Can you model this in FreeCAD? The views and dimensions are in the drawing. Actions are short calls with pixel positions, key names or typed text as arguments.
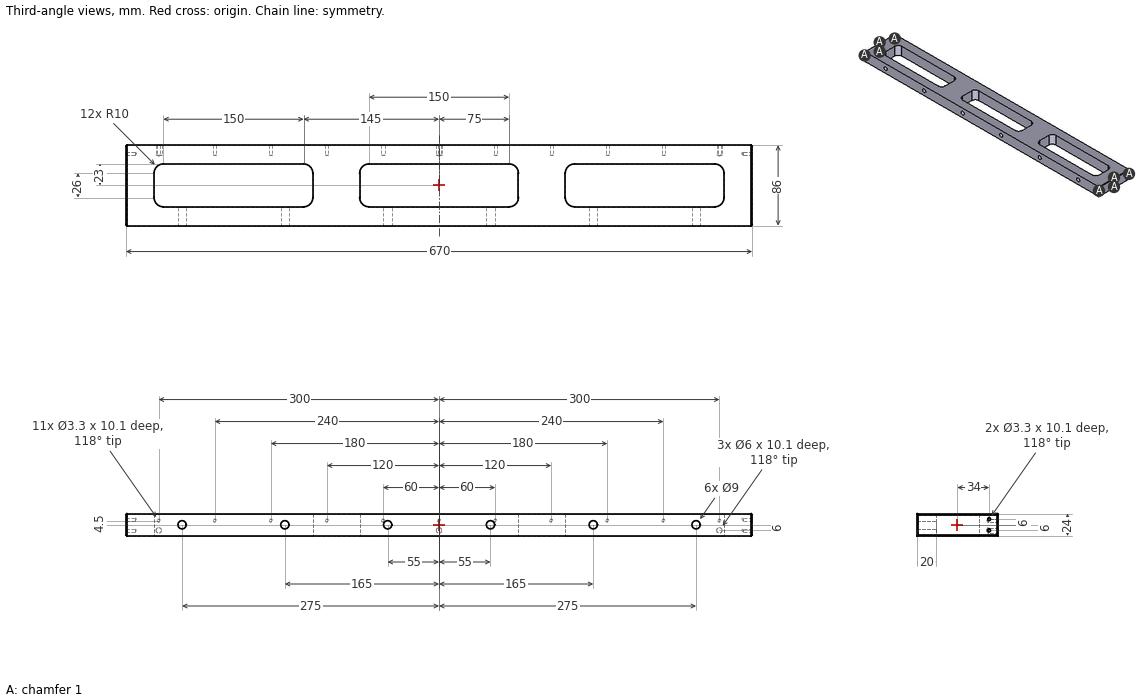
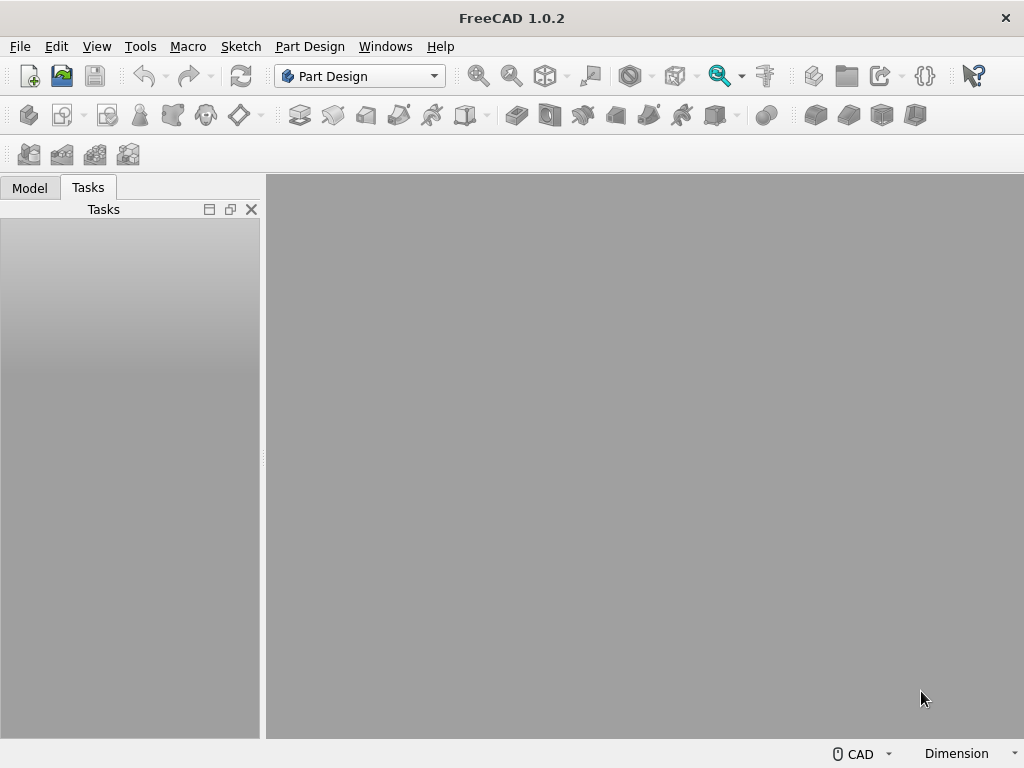
key(ctrl+n)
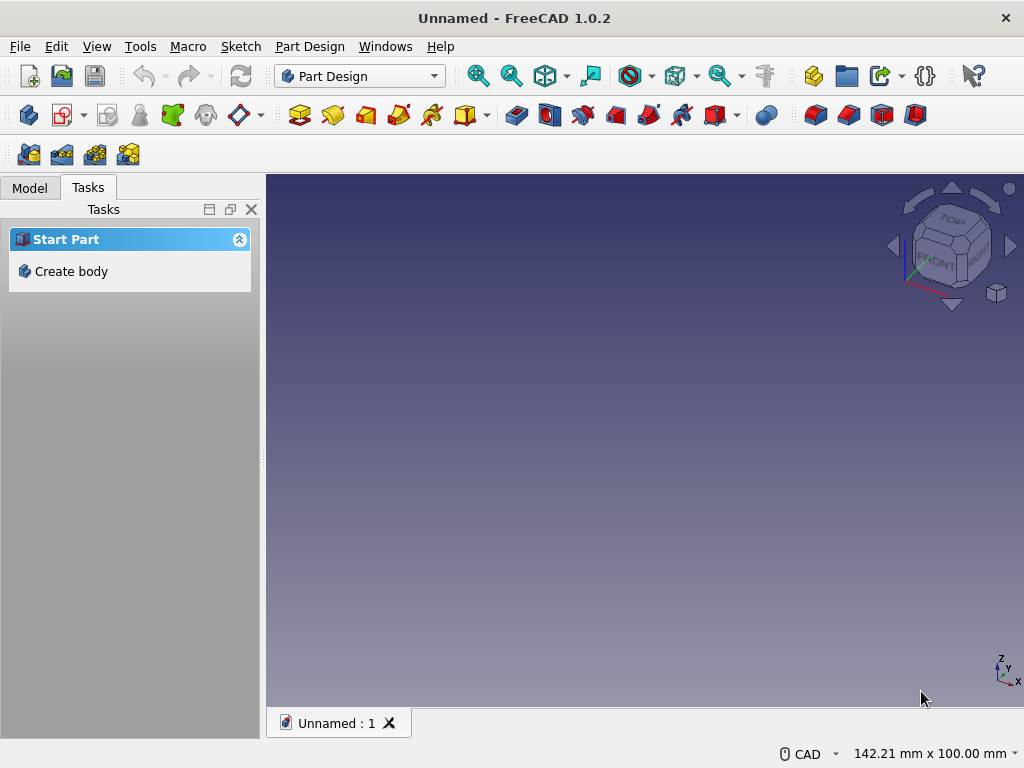
click(62, 116)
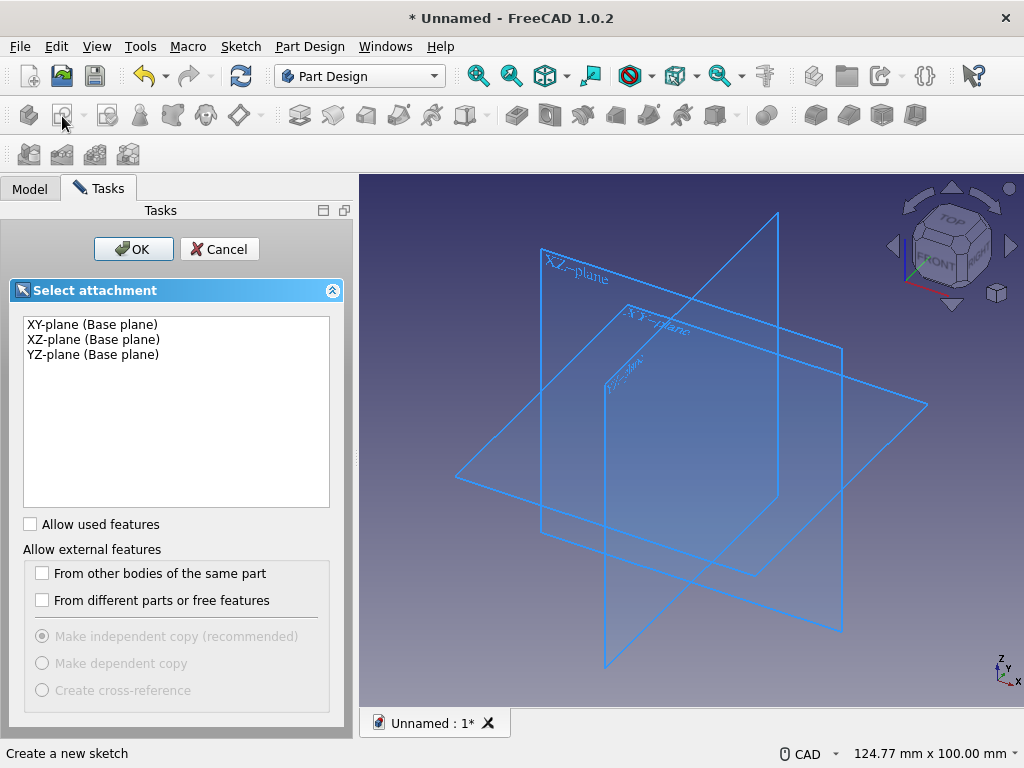
click(84, 324)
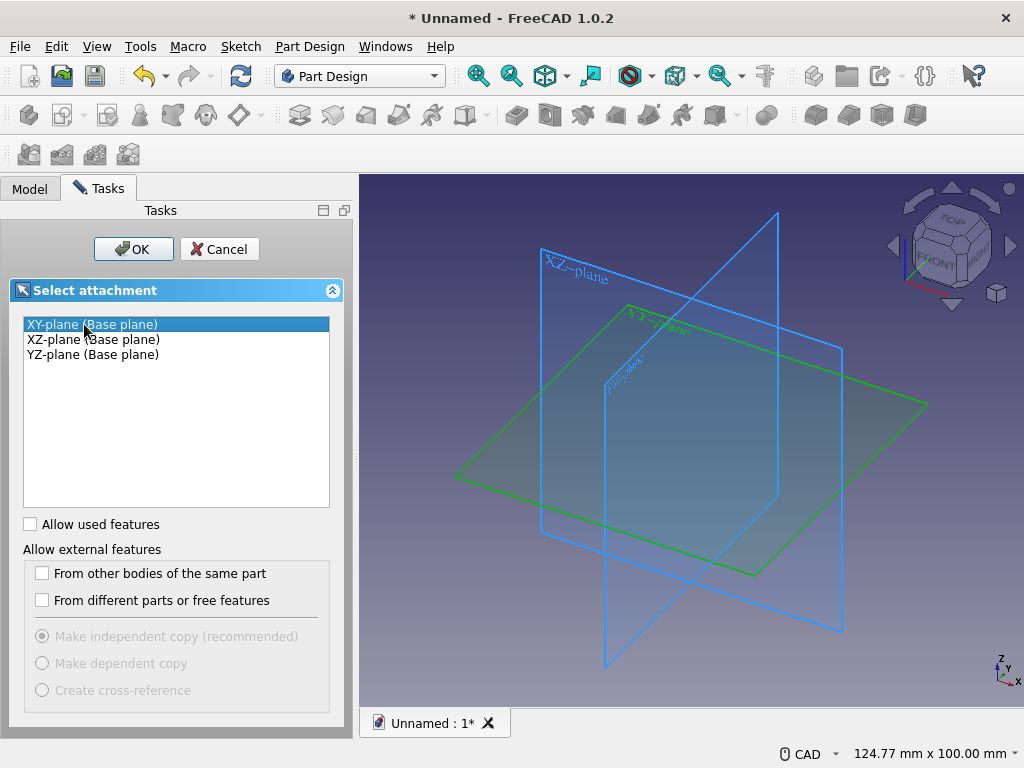
click(134, 249)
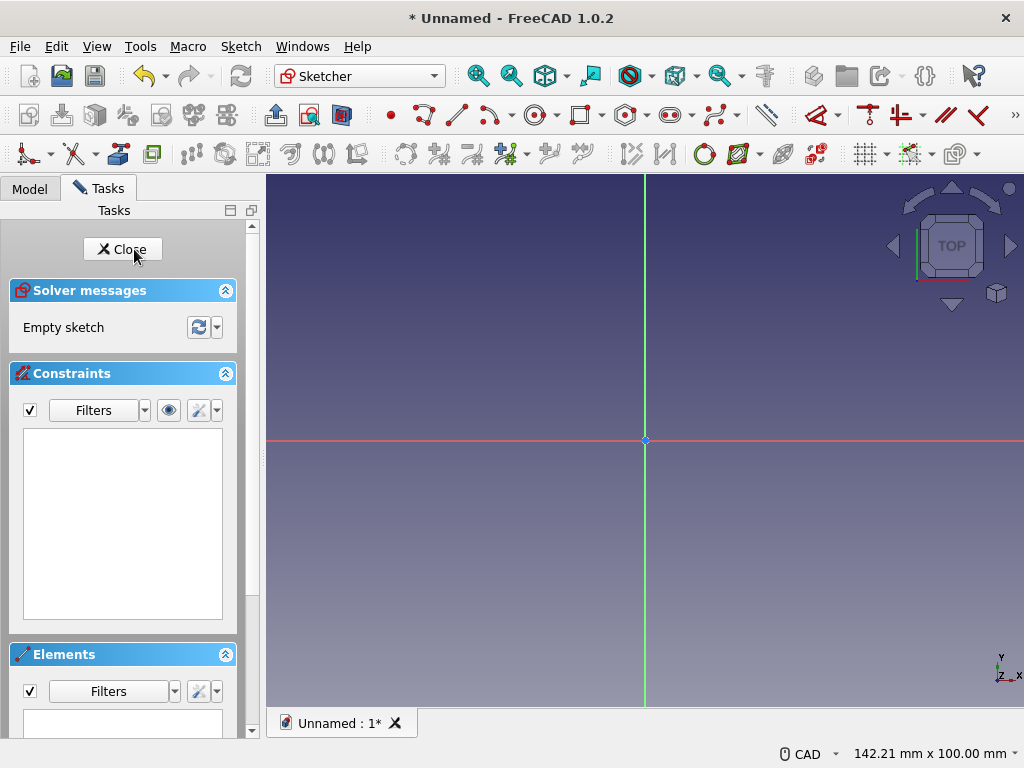
scroll(568, 441, down, 11)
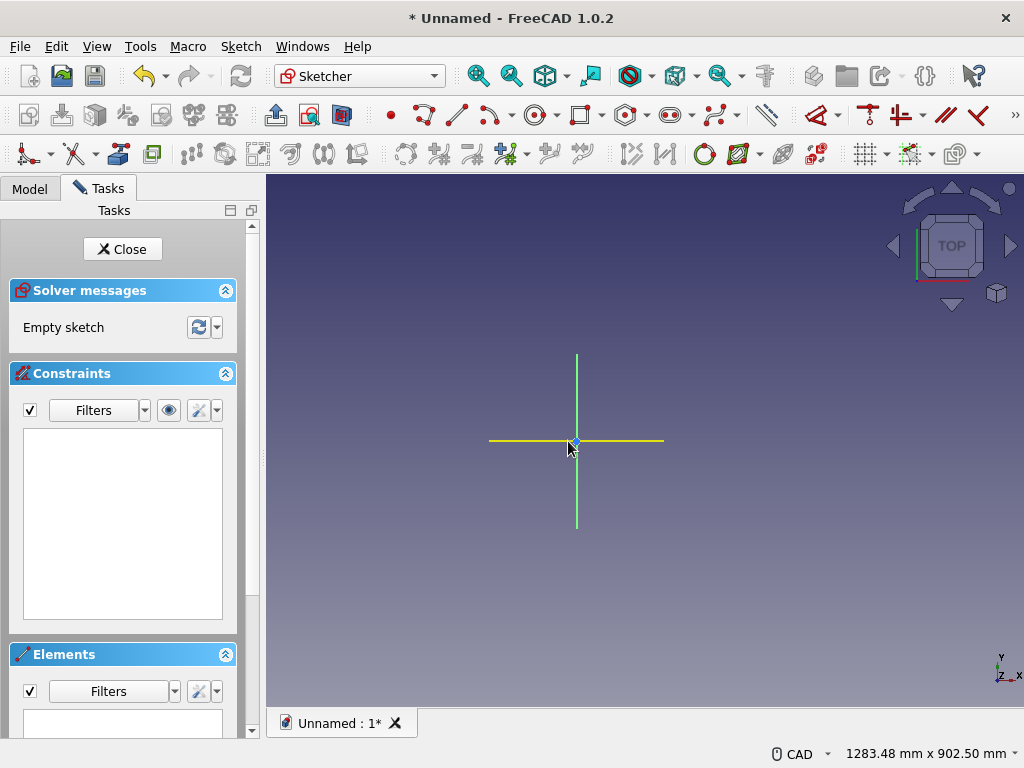
key(g)
key(v)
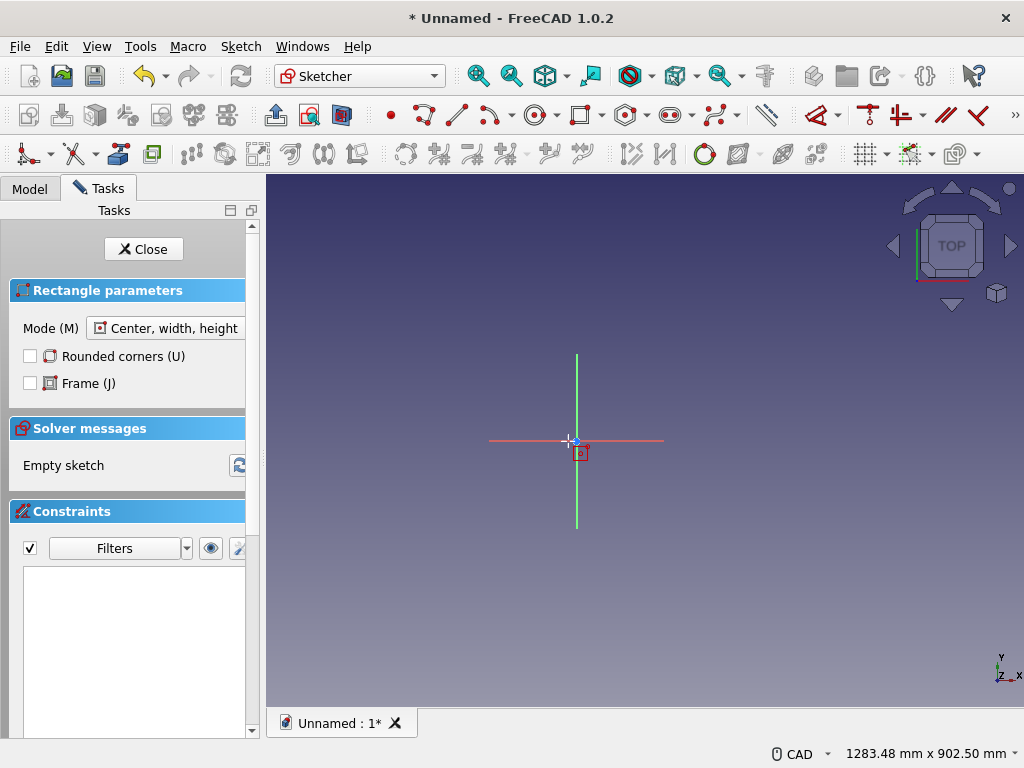
click(577, 441)
move(775, 416)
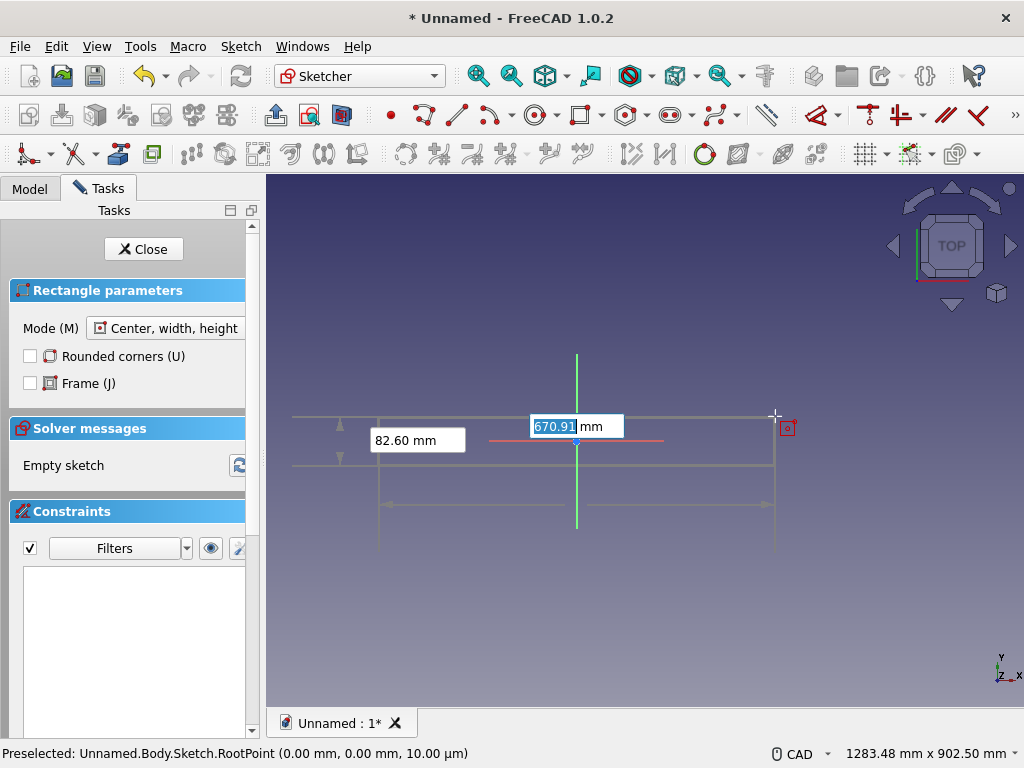
text(670)
key(Tab)
text(86)
key(Return)
key(Escape)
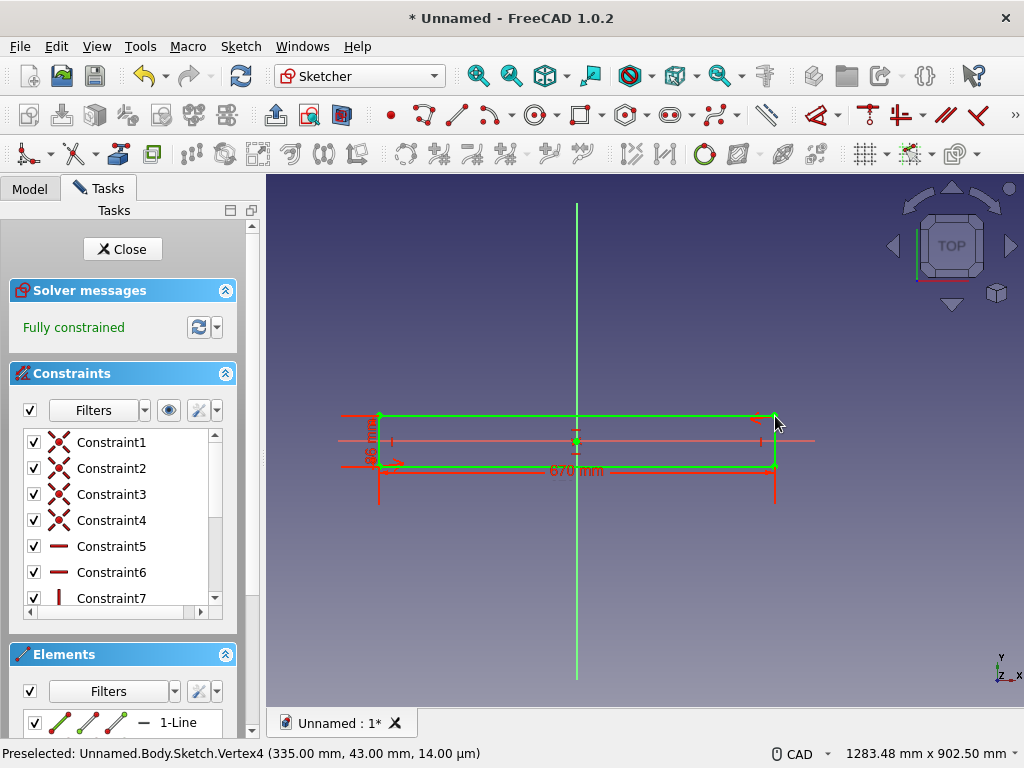
click(123, 249)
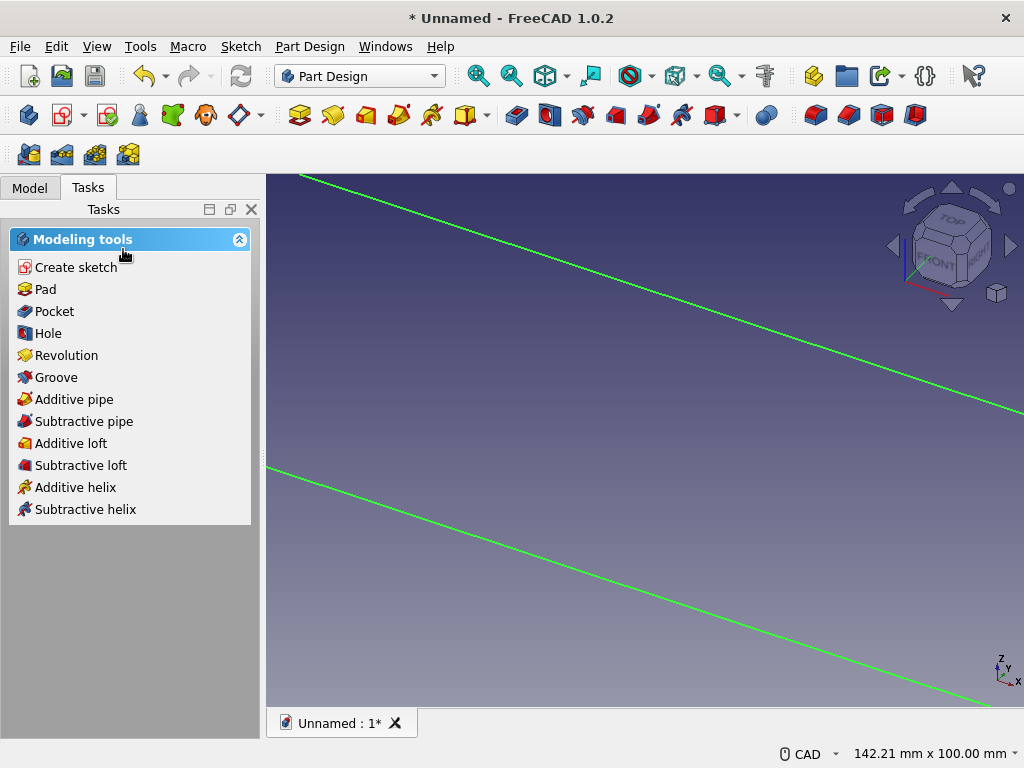
click(300, 116)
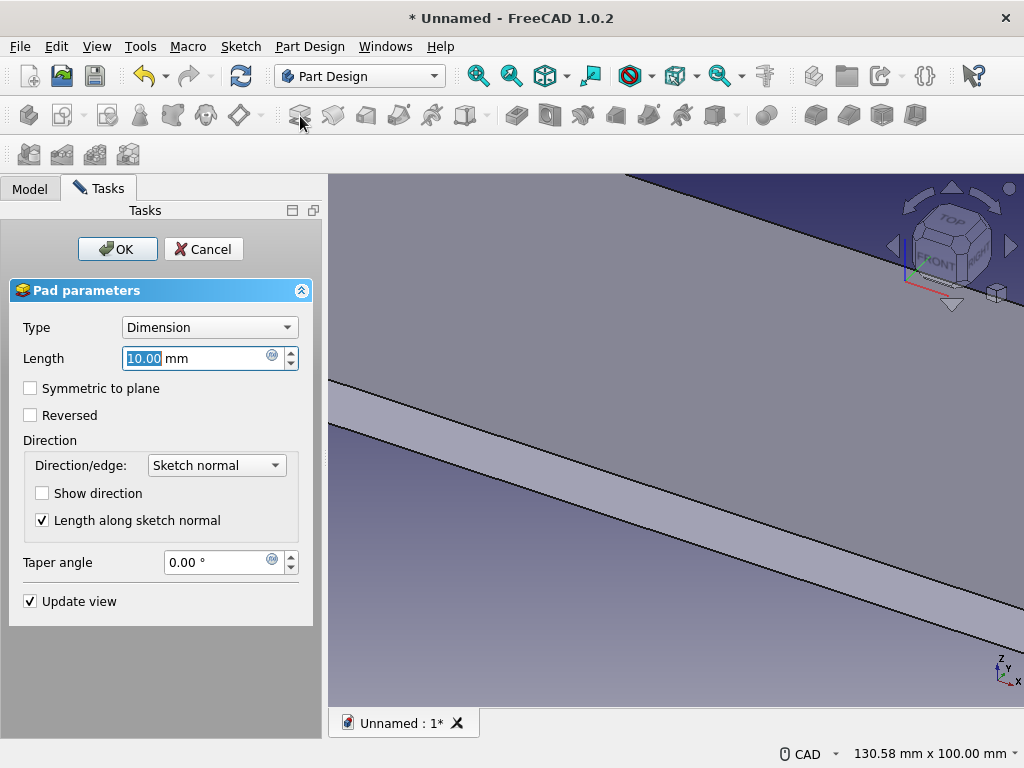
text(24)
key(Tab)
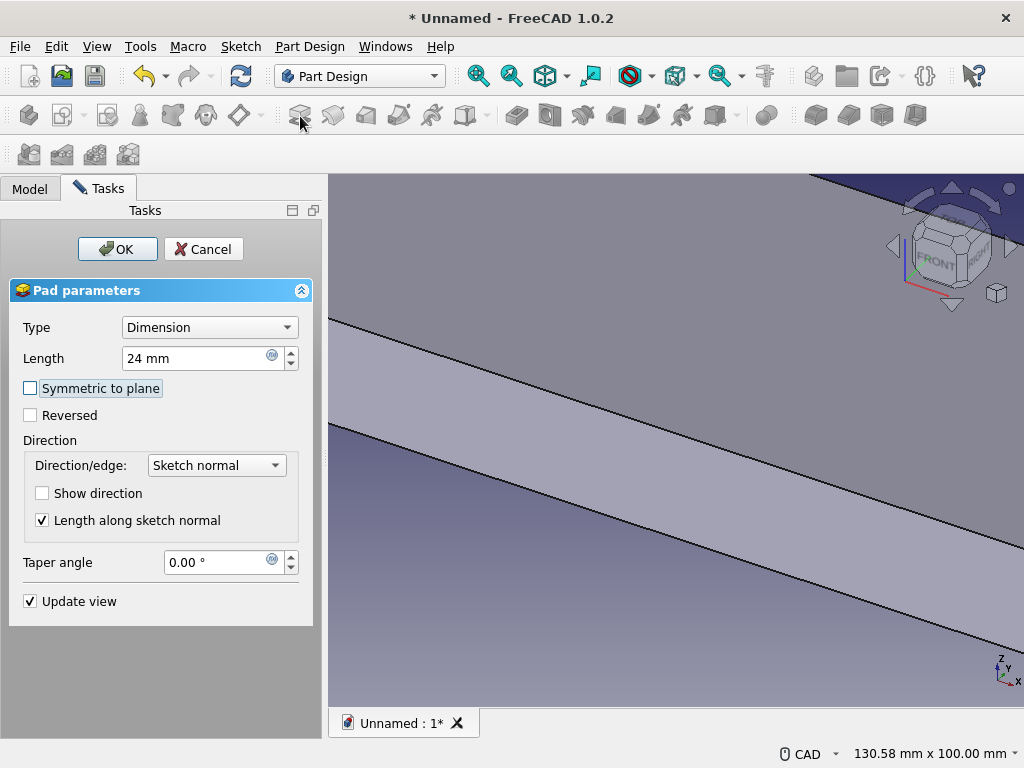
click(31, 388)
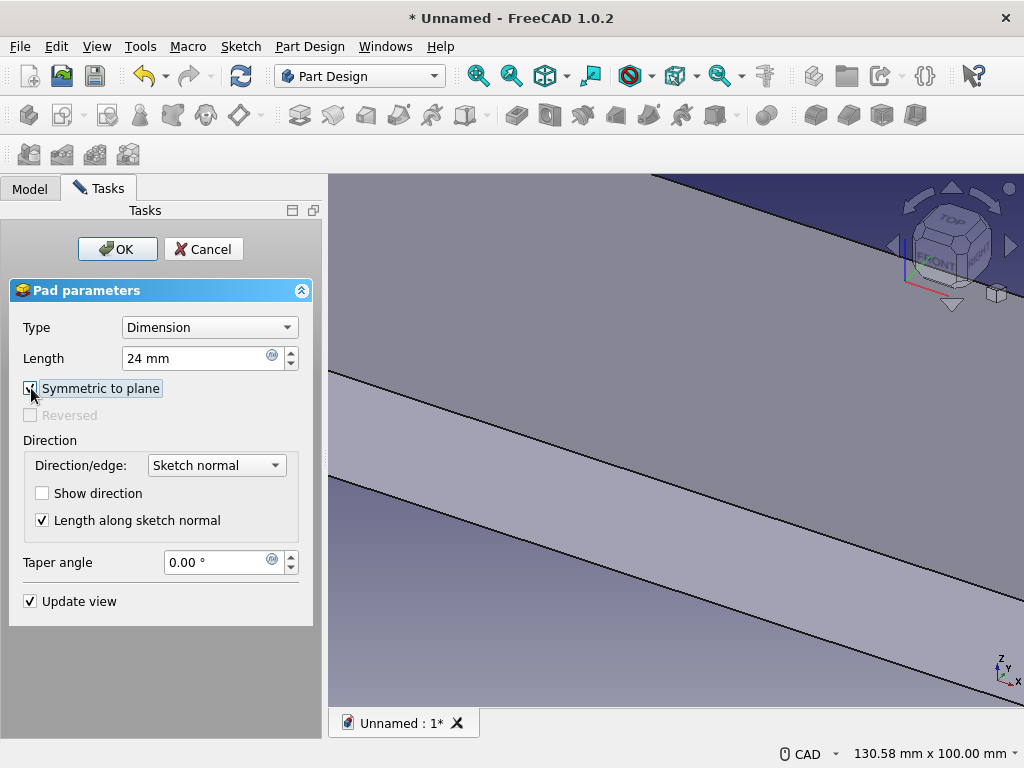
click(118, 249)